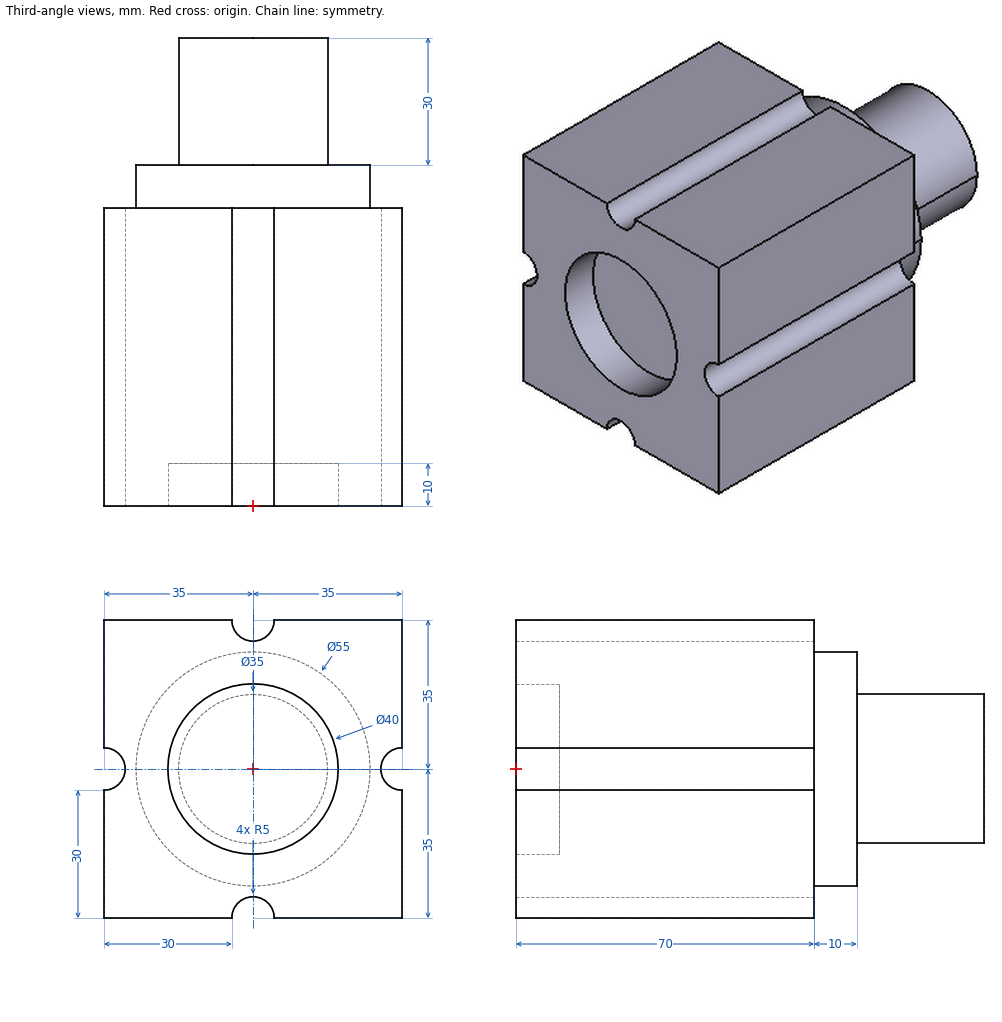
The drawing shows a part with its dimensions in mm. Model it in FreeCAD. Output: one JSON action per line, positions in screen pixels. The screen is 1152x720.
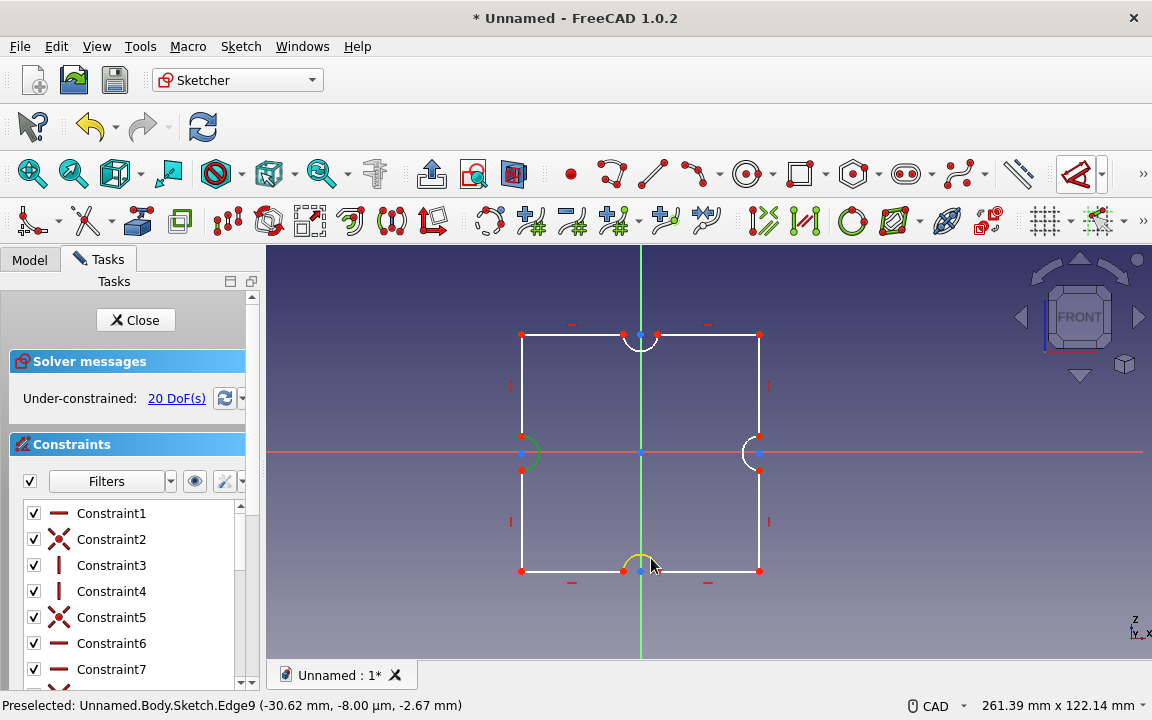
{"action": "scroll", "coordinate": [631, 348], "scroll_direction": "up", "scroll_amount": 2}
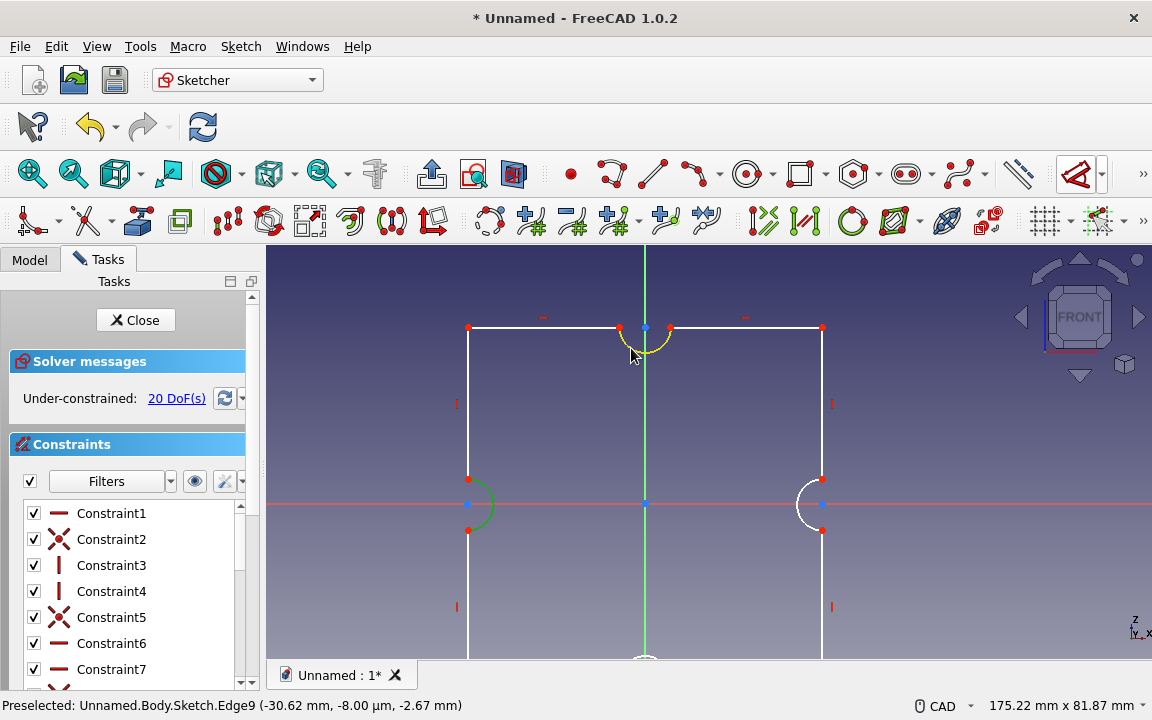
{"action": "left_click", "coordinate": [630, 348]}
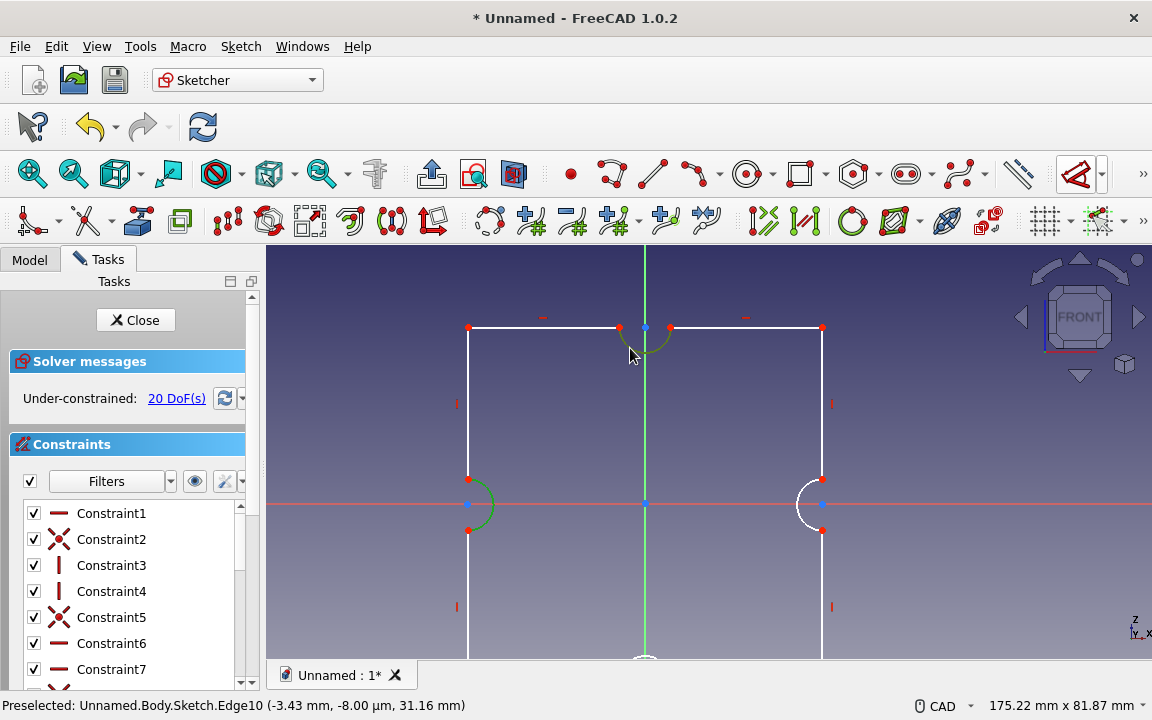
{"action": "left_click", "coordinate": [802, 490]}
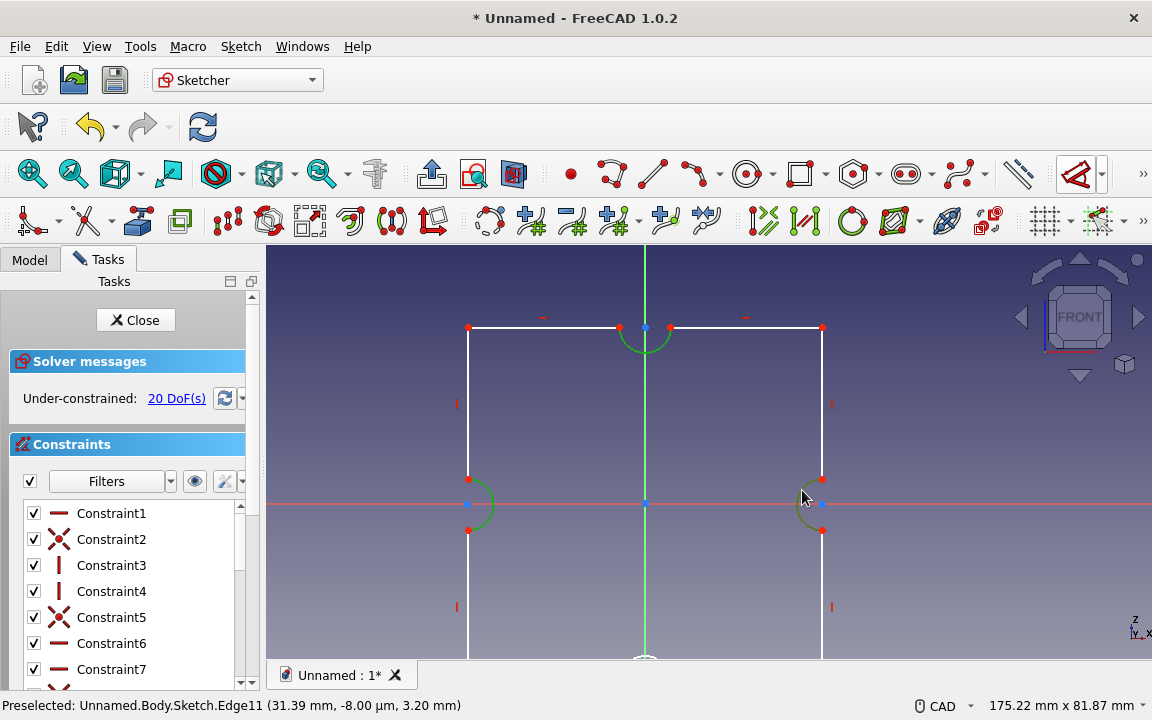
{"action": "scroll", "coordinate": [631, 347], "scroll_direction": "down", "scroll_amount": 2}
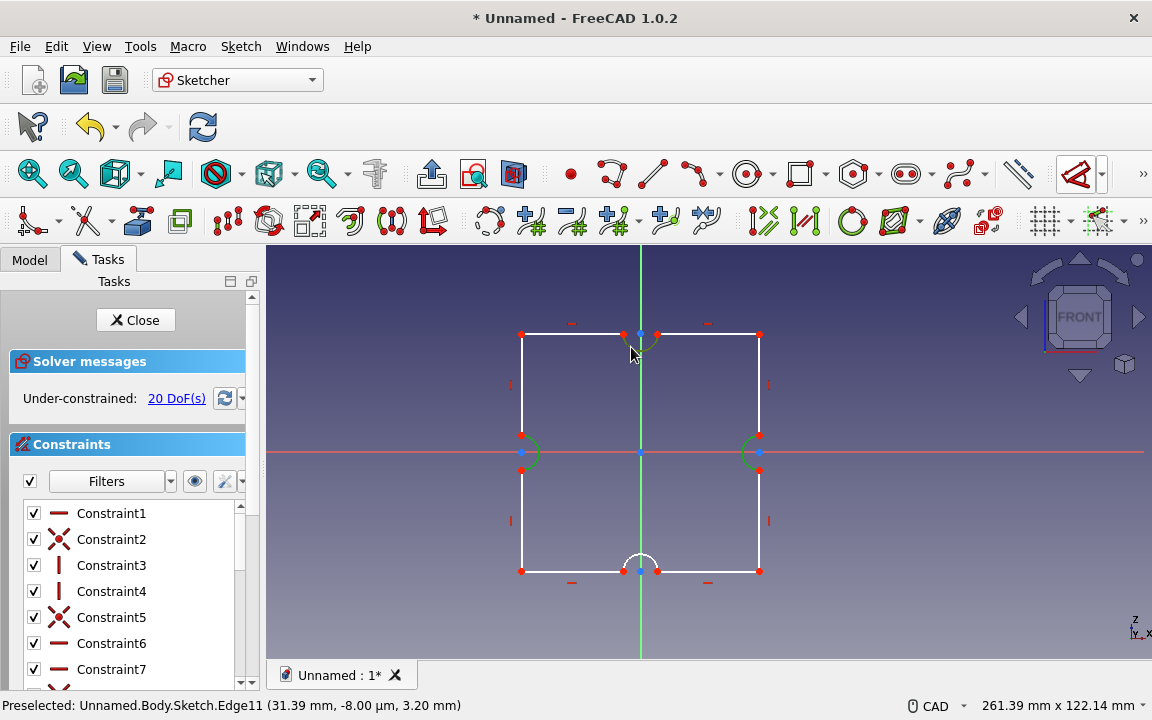
{"action": "scroll", "coordinate": [651, 558], "scroll_direction": "up", "scroll_amount": 2}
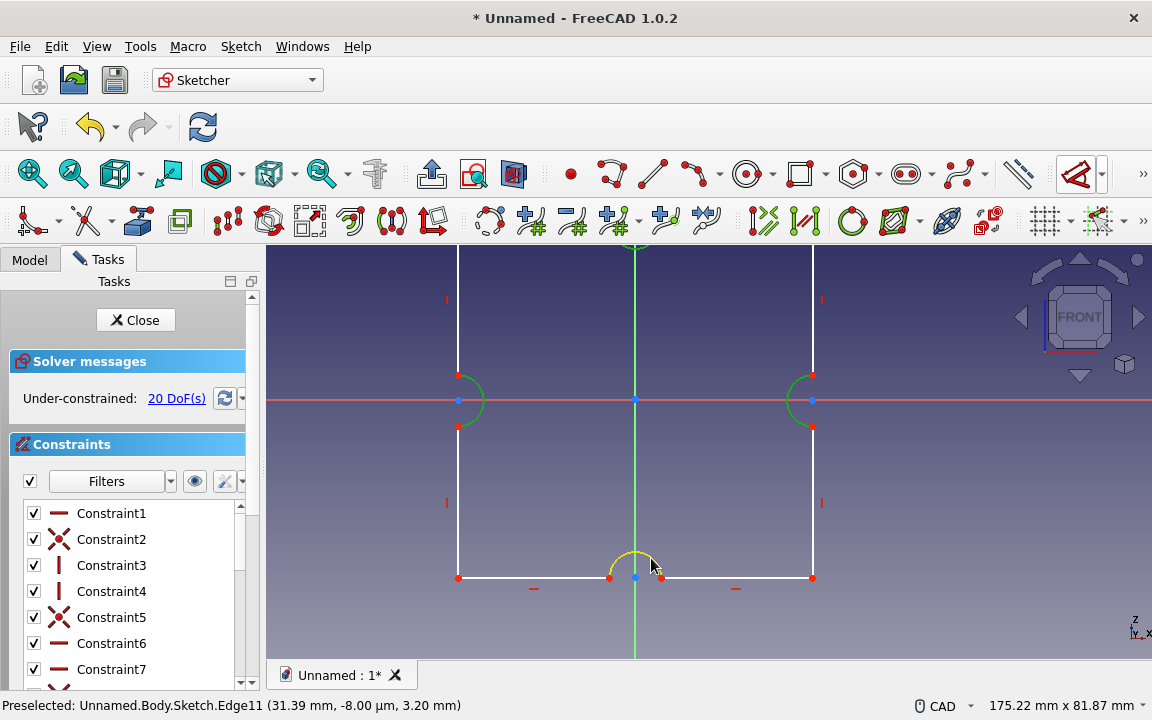
{"action": "left_click", "coordinate": [651, 557]}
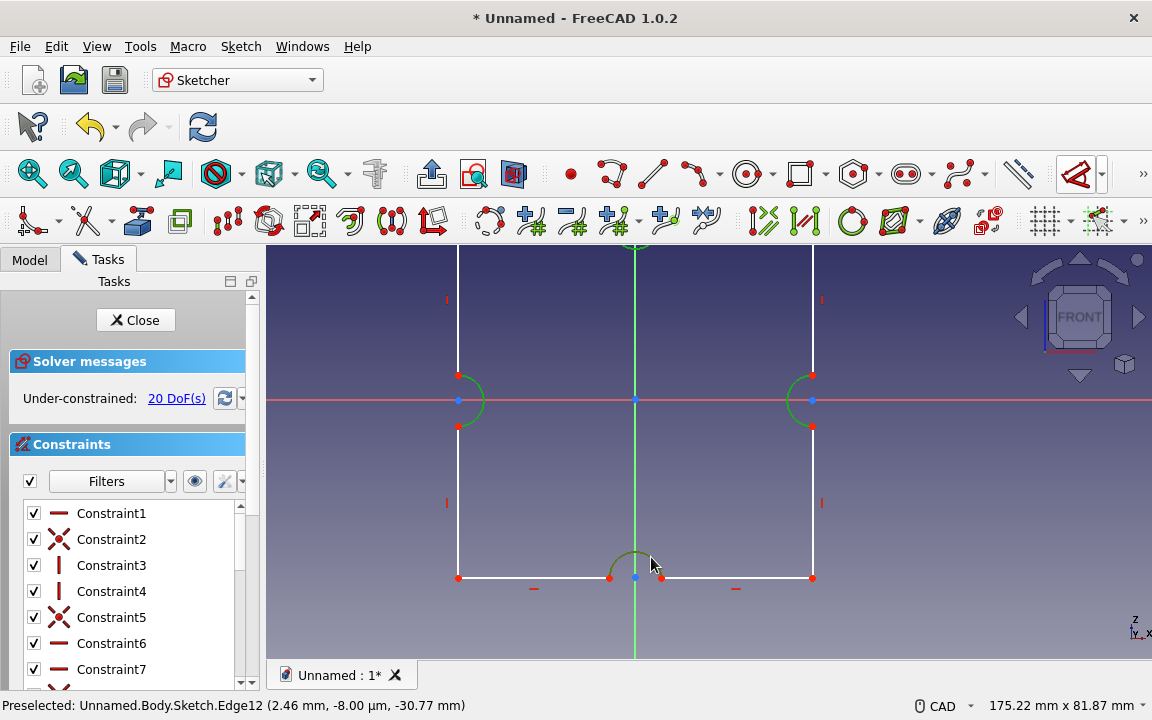
{"action": "key", "text": "e"}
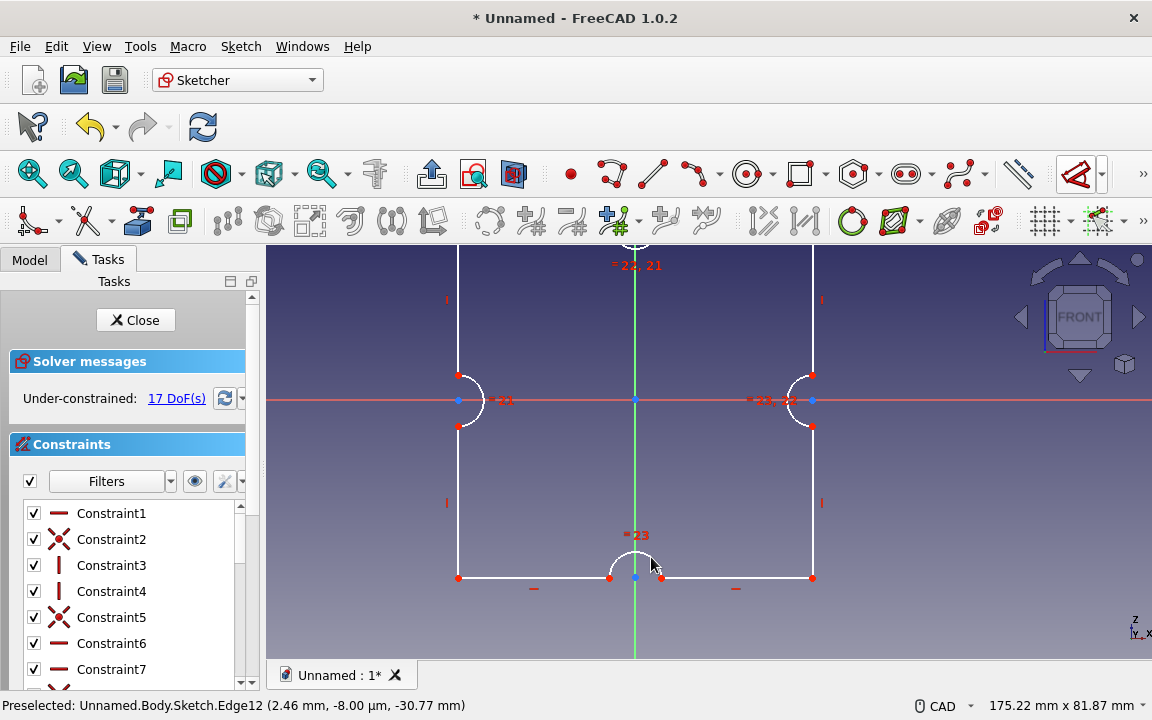
{"action": "left_click", "coordinate": [458, 401]}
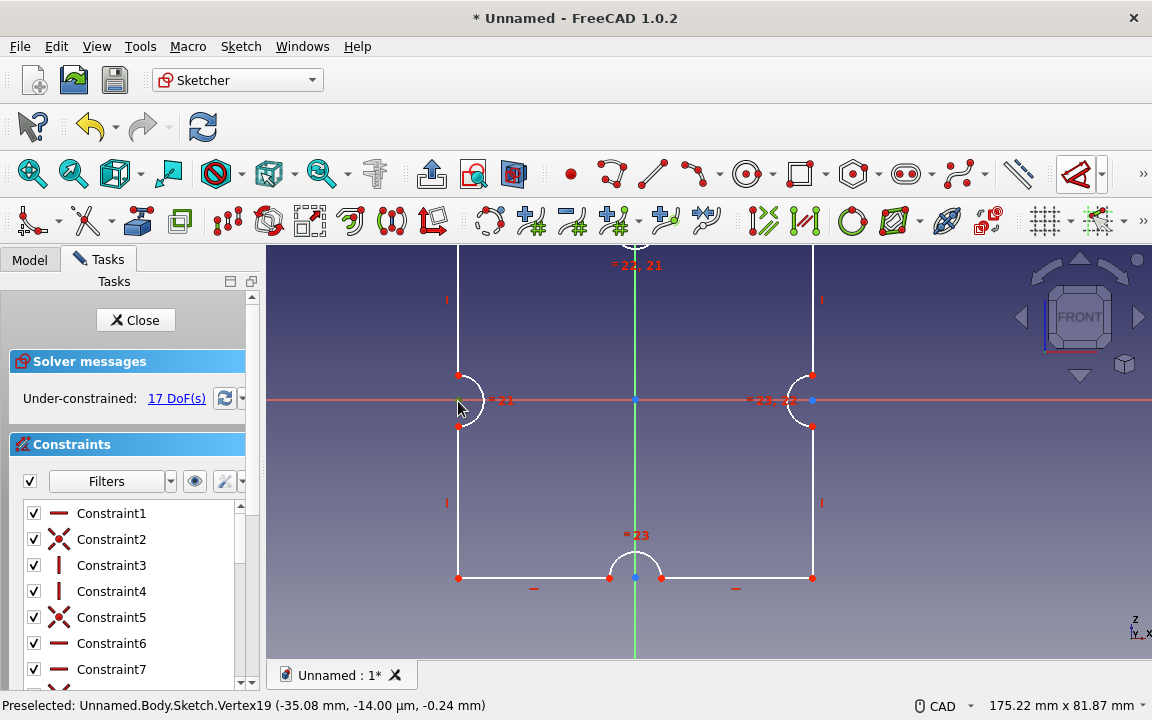
{"action": "left_click", "coordinate": [343, 400]}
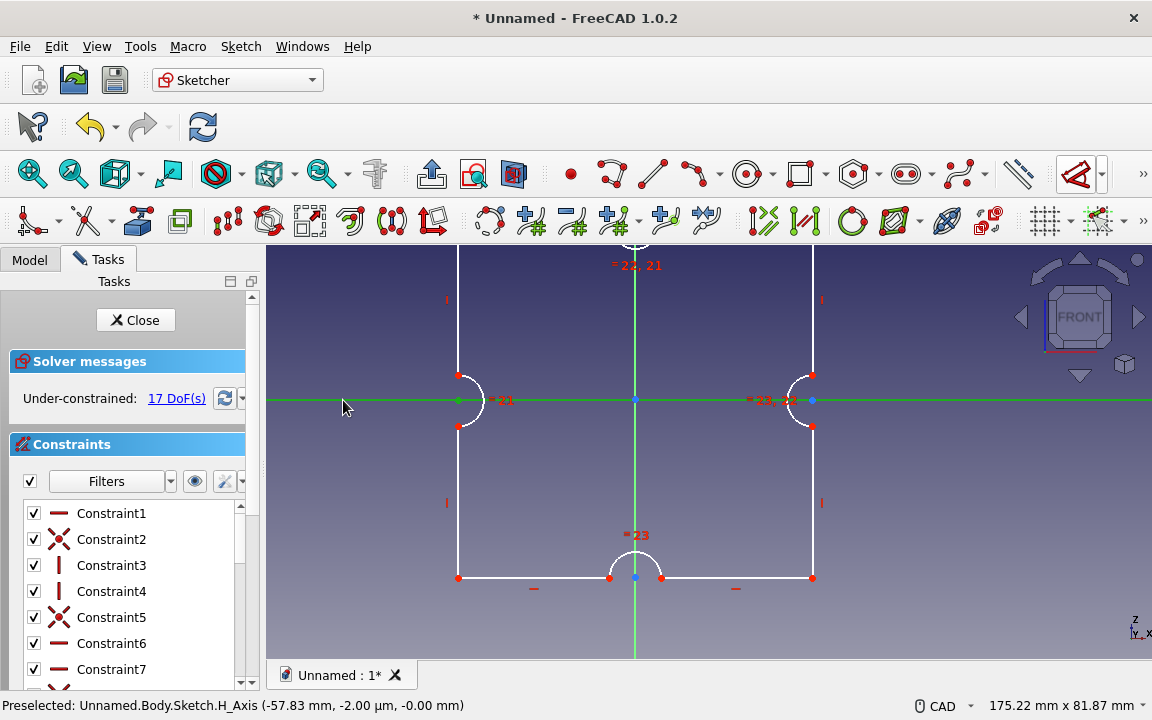
{"action": "key", "text": "c"}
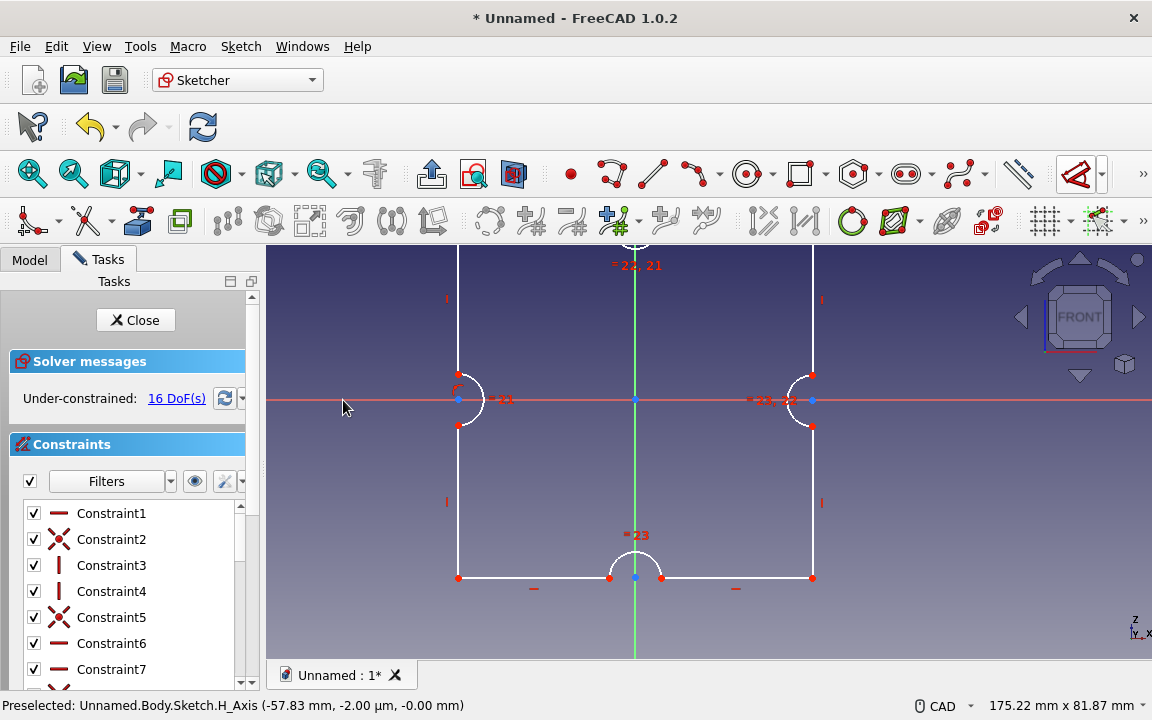
{"action": "scroll", "coordinate": [651, 558], "scroll_direction": "down", "scroll_amount": 2}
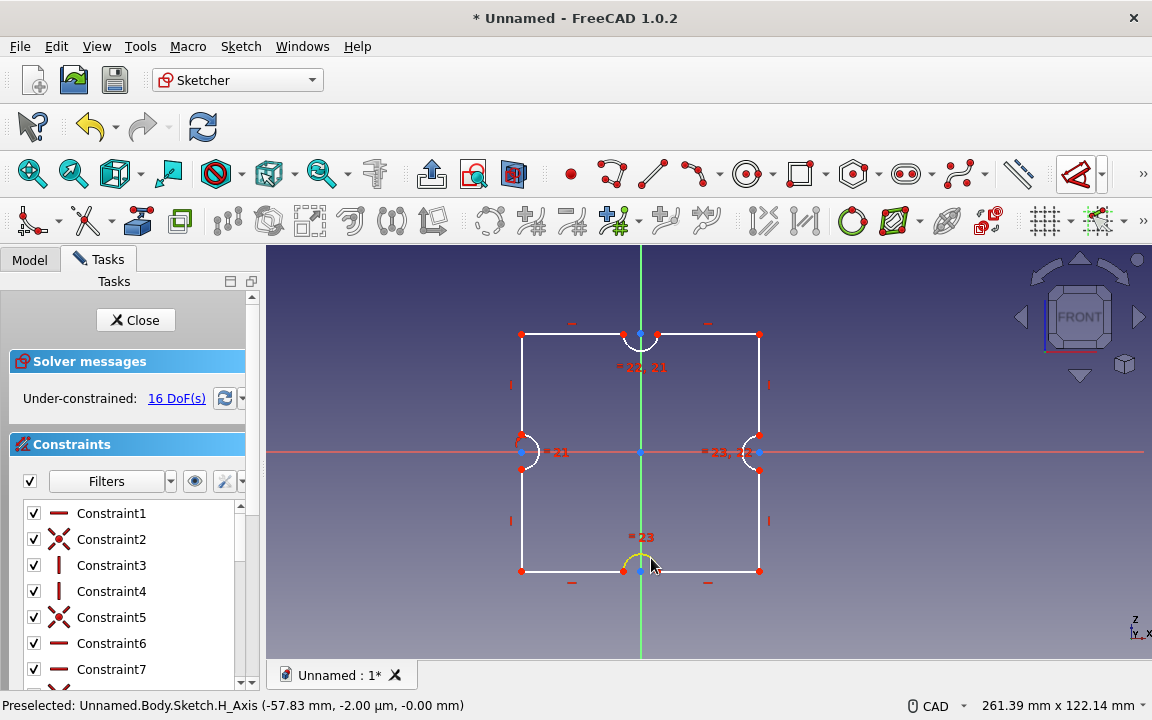
{"action": "left_click", "coordinate": [641, 334]}